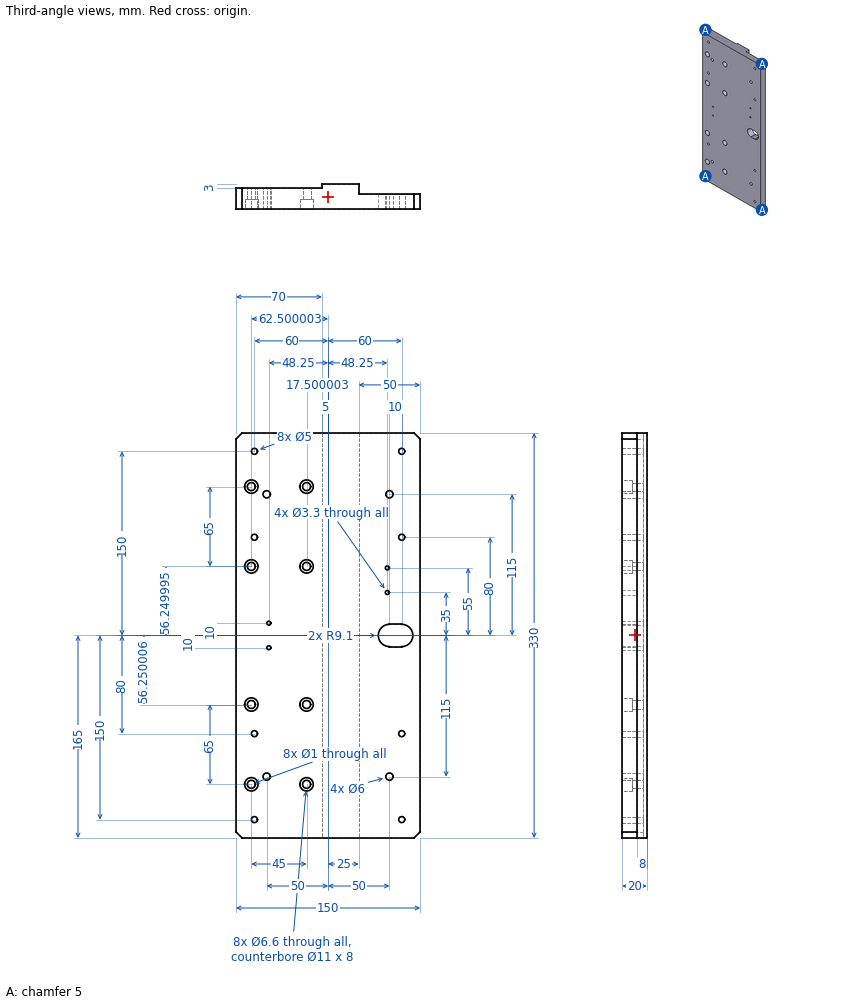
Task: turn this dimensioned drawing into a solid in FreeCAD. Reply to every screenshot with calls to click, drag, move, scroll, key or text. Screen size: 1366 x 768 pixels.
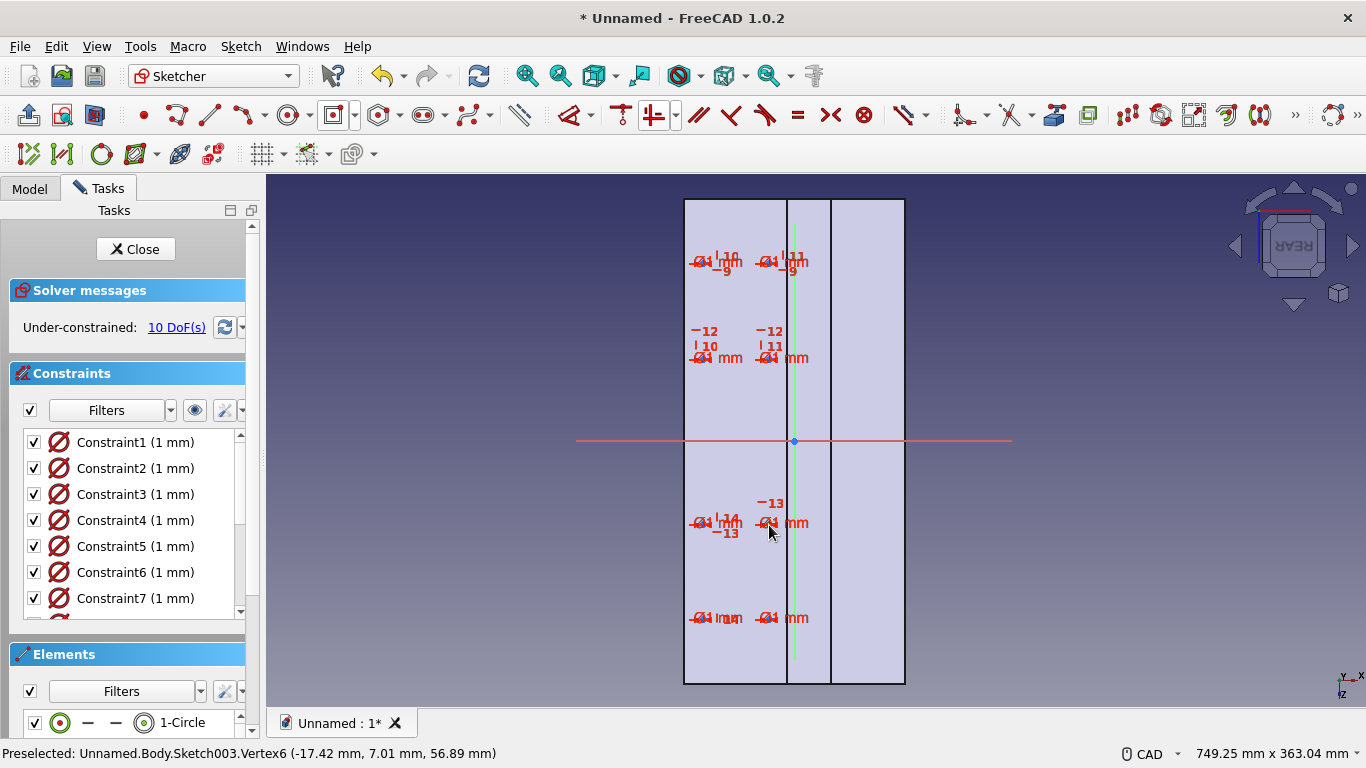
click(769, 620)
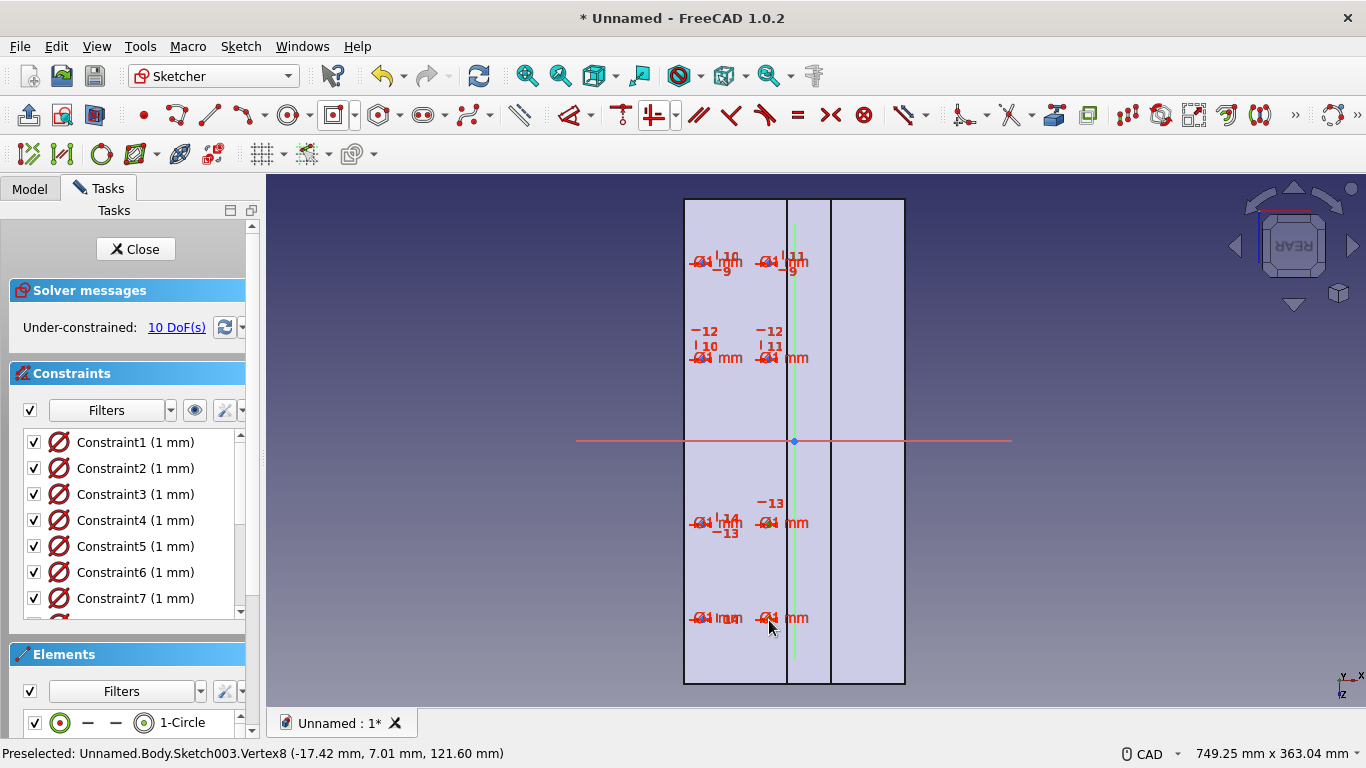
click(676, 116)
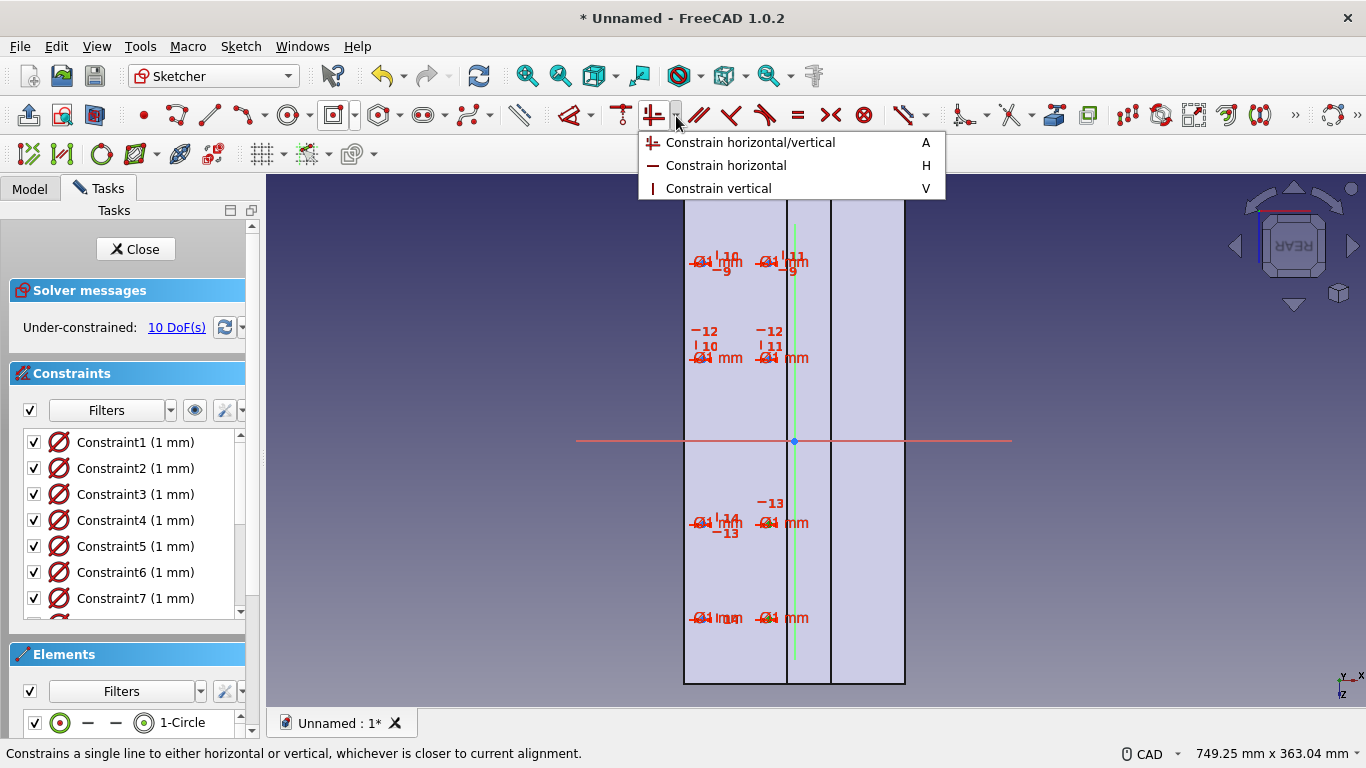
click(792, 188)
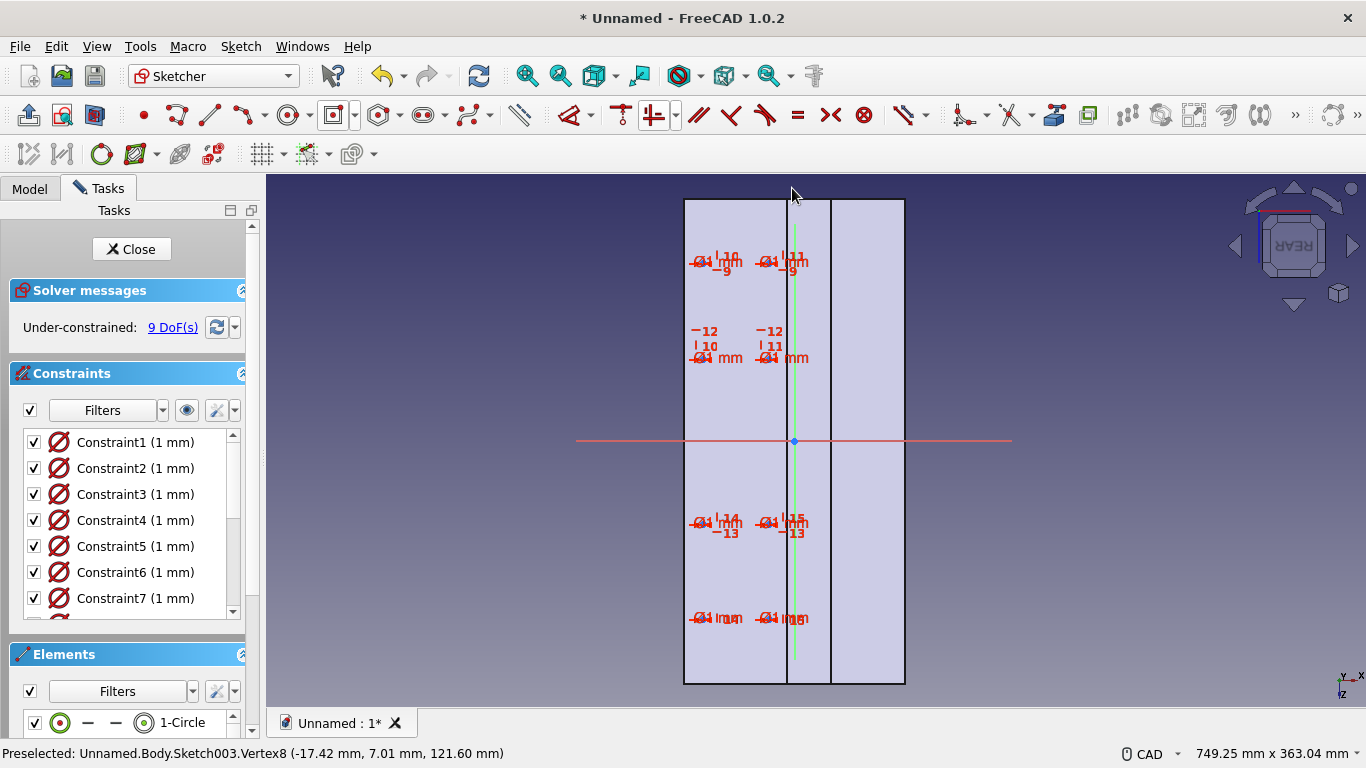
click(703, 620)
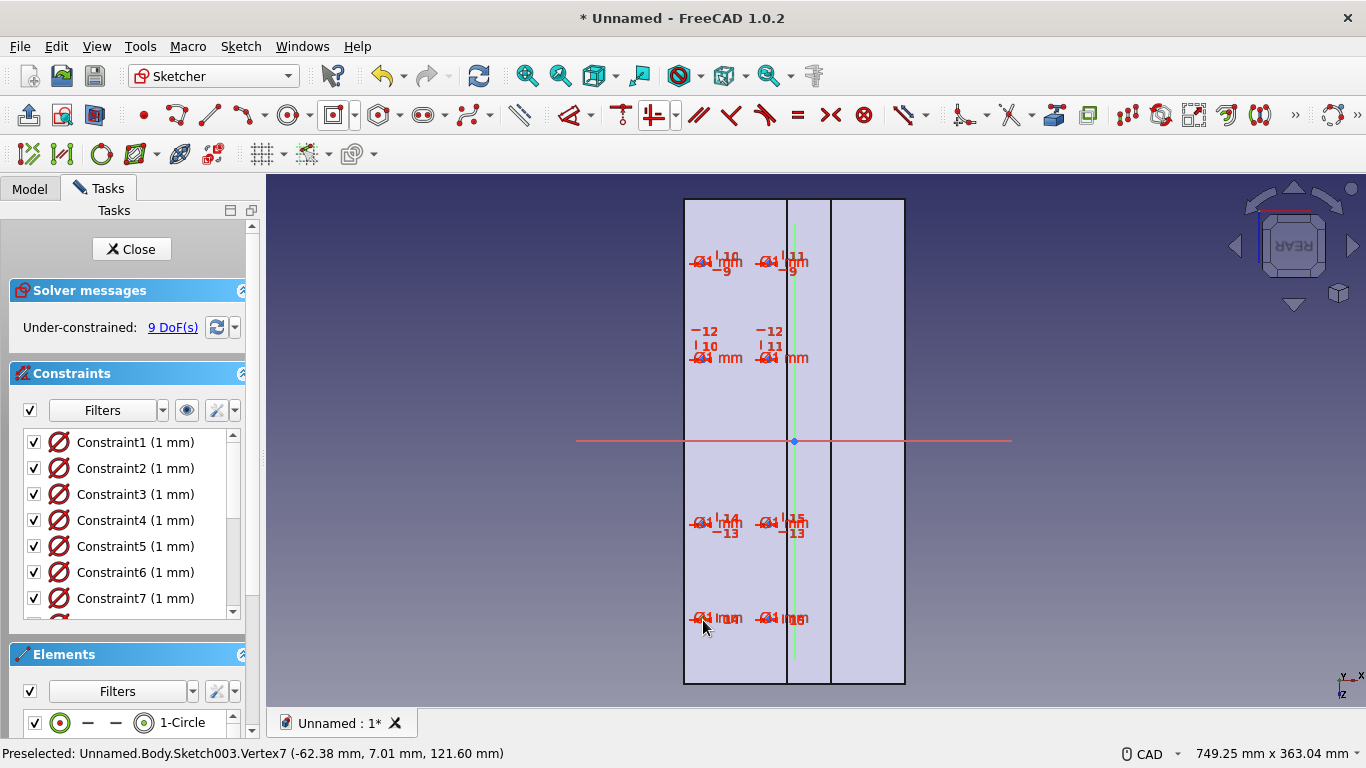
click(769, 620)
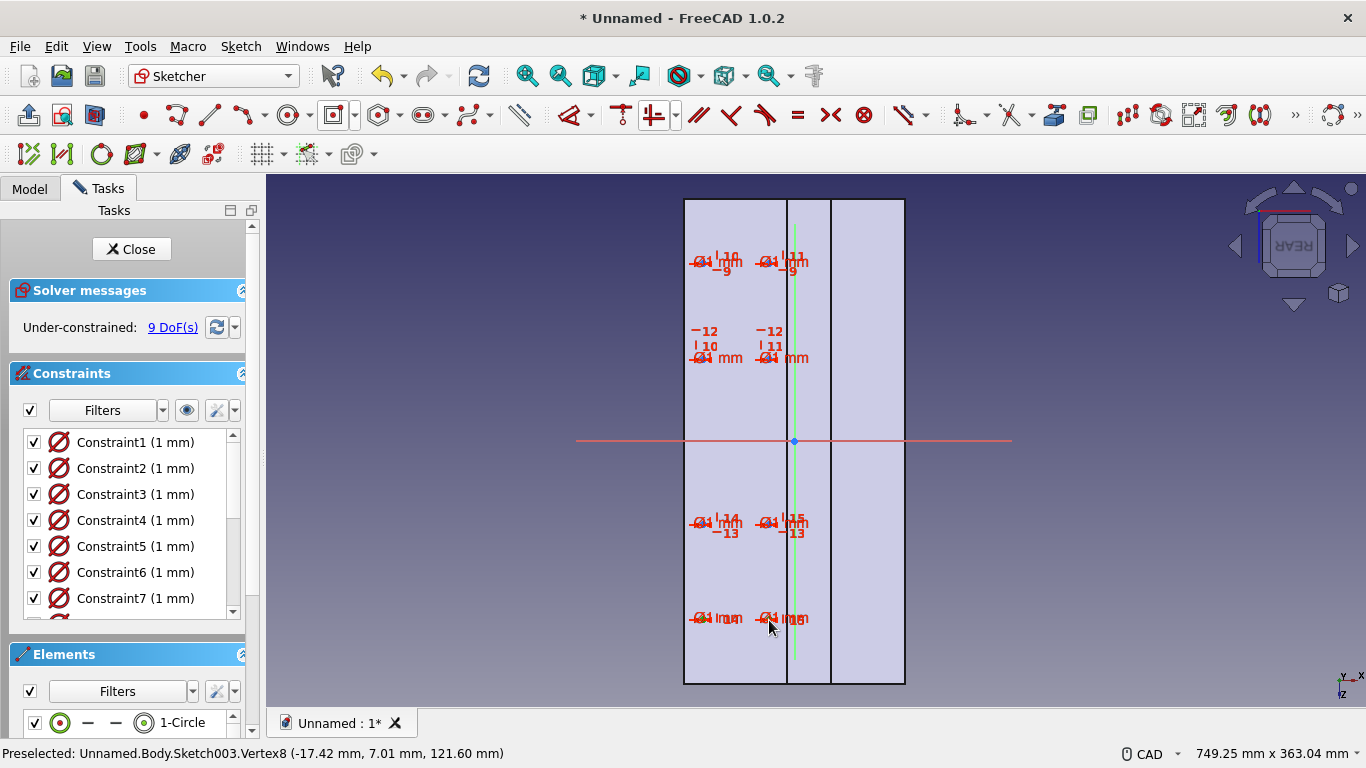
click(676, 116)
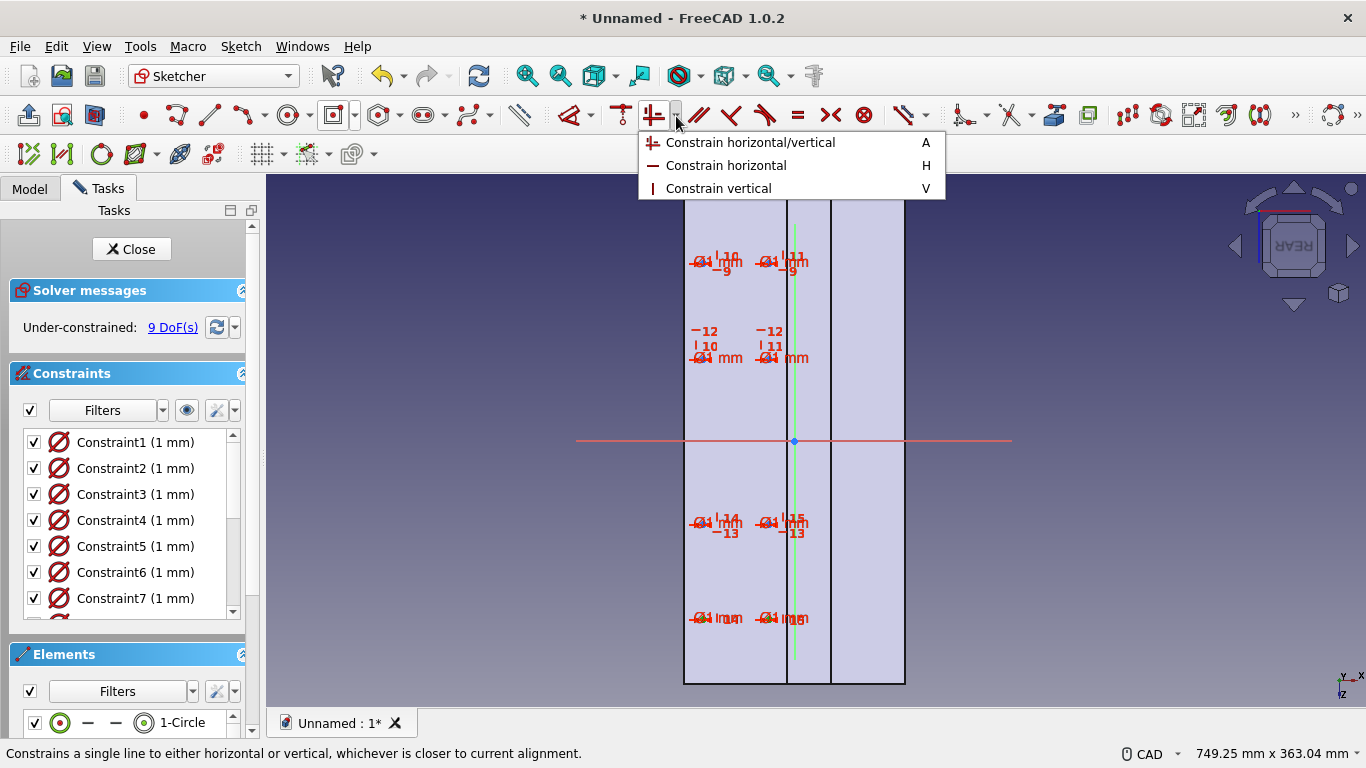
click(792, 166)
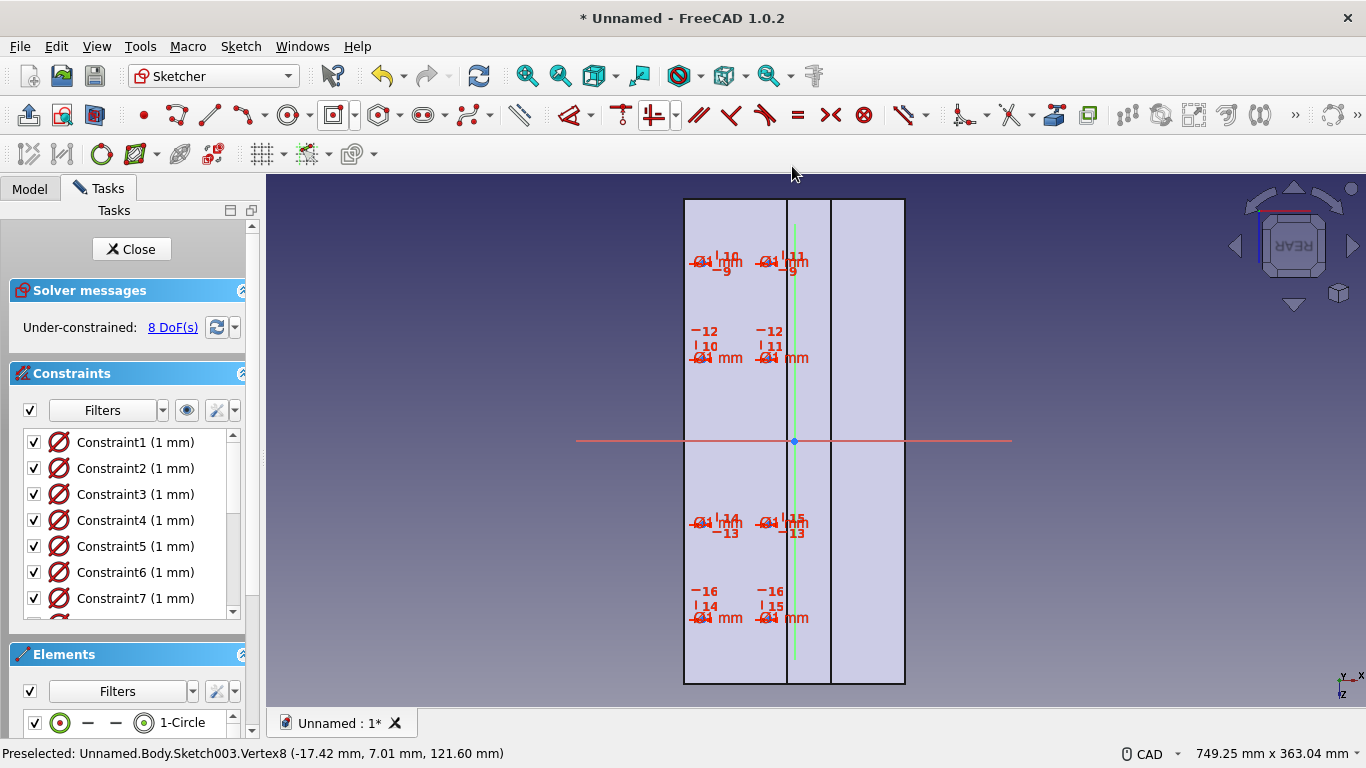
click(568, 116)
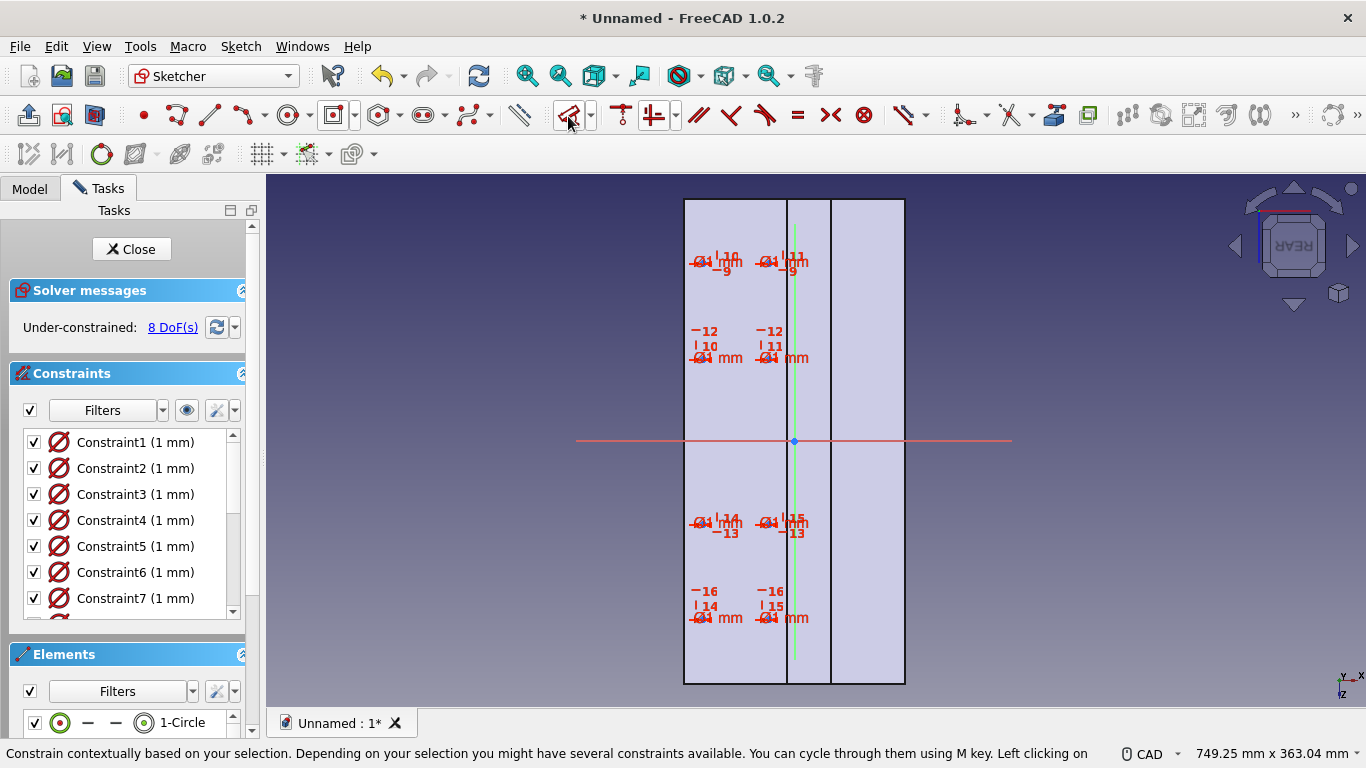
click(703, 264)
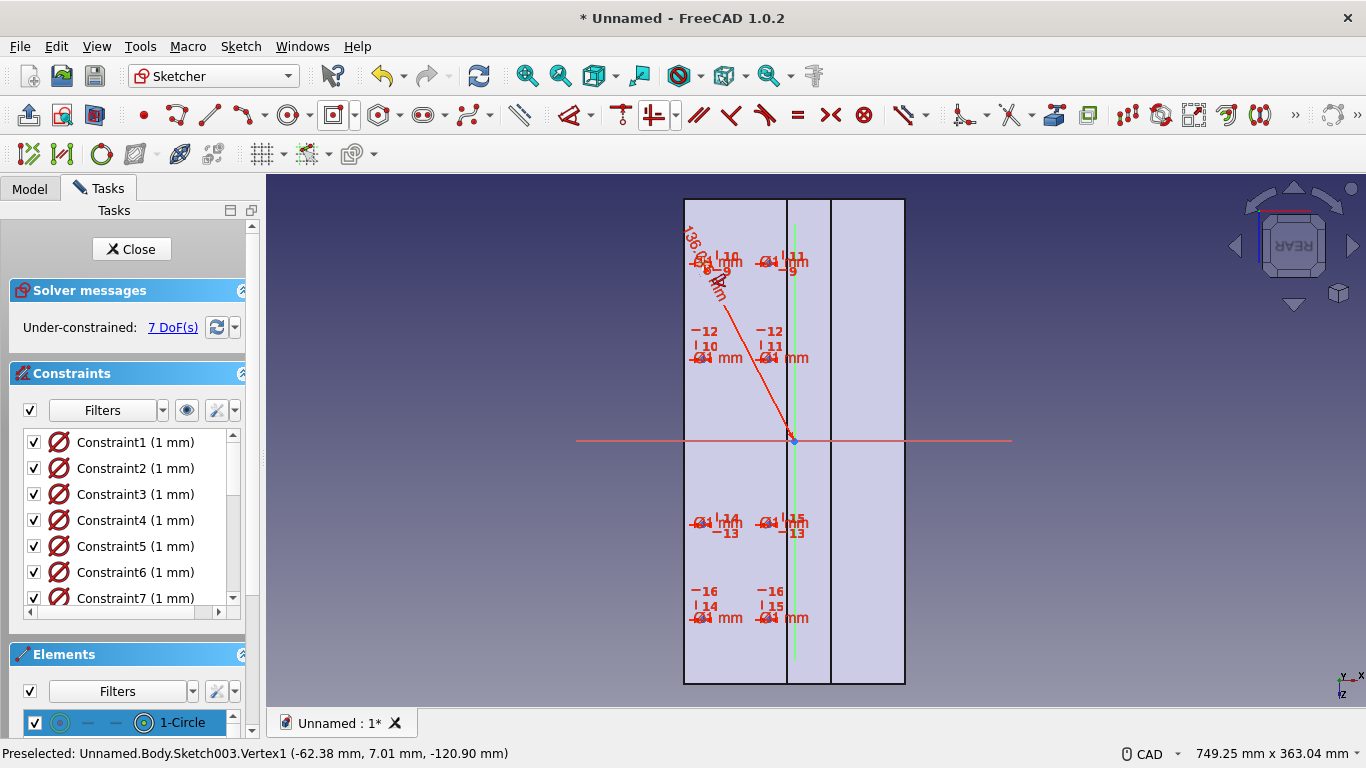
click(769, 264)
click(736, 230)